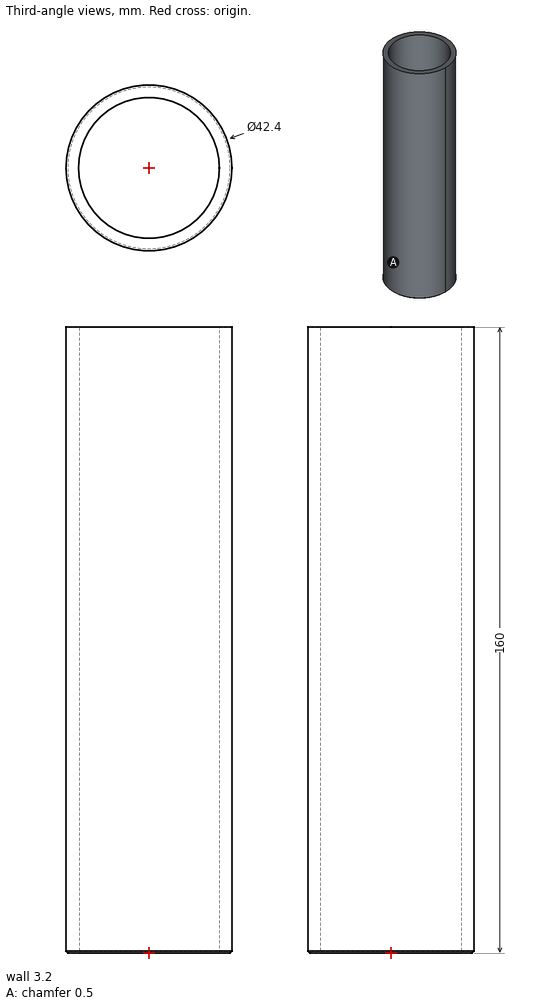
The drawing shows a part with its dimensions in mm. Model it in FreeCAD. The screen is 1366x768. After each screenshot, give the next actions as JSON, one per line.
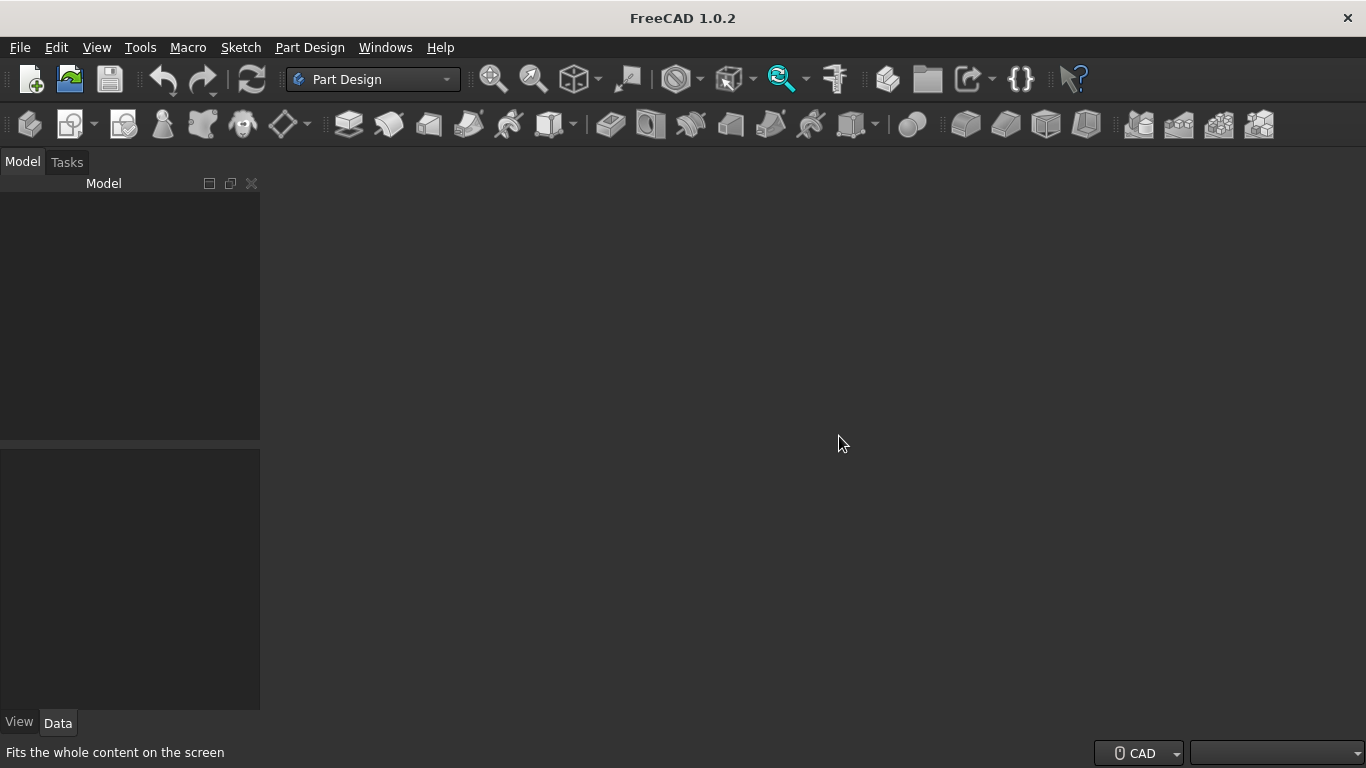
{"action": "left_click", "coordinate": [30, 80]}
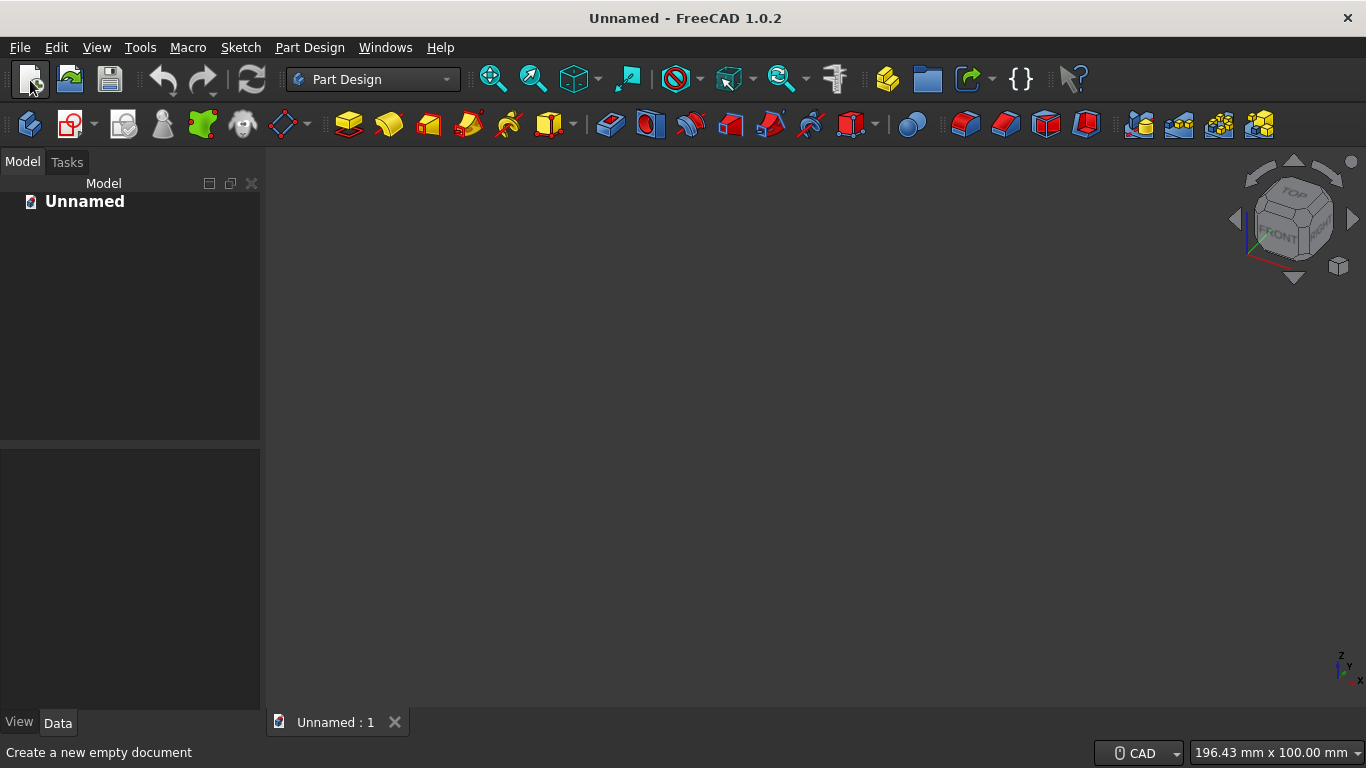
{"action": "left_click", "coordinate": [70, 124]}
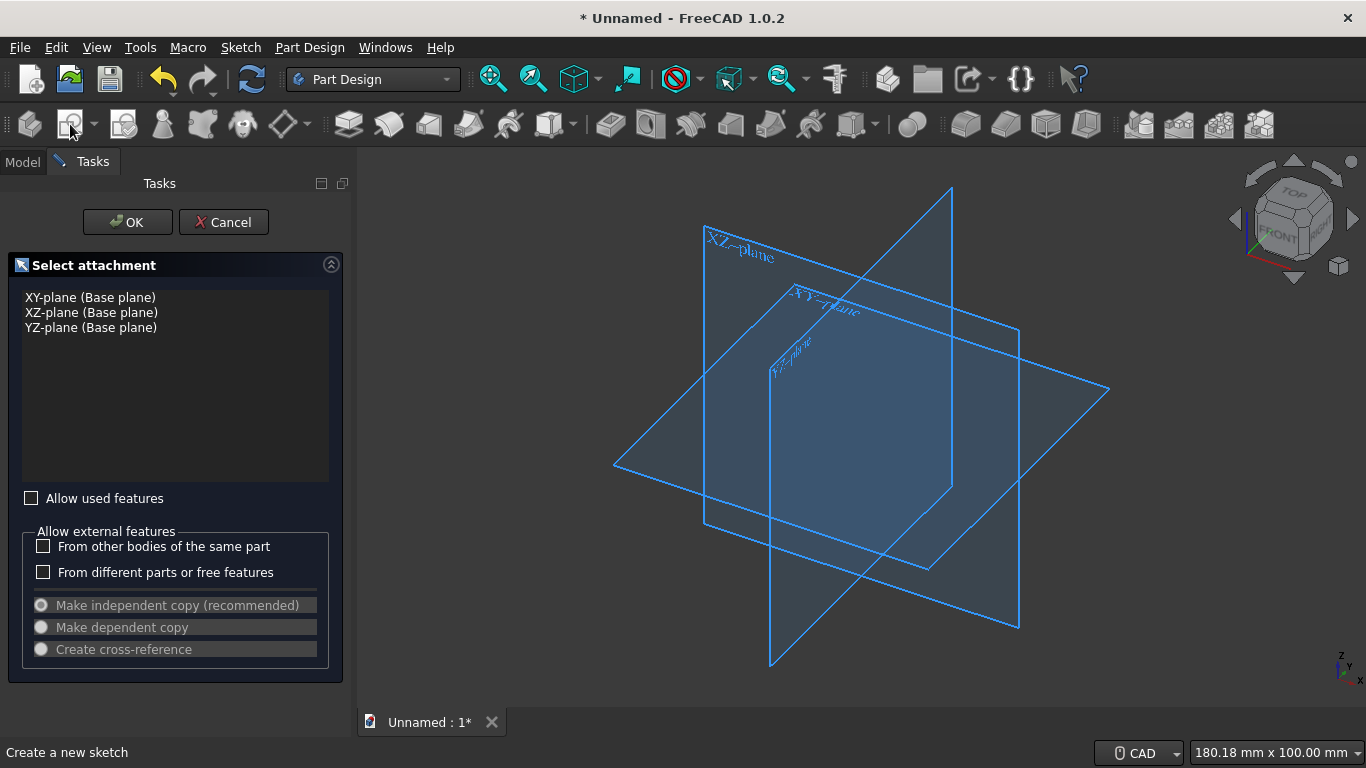
{"action": "left_click", "coordinate": [82, 298]}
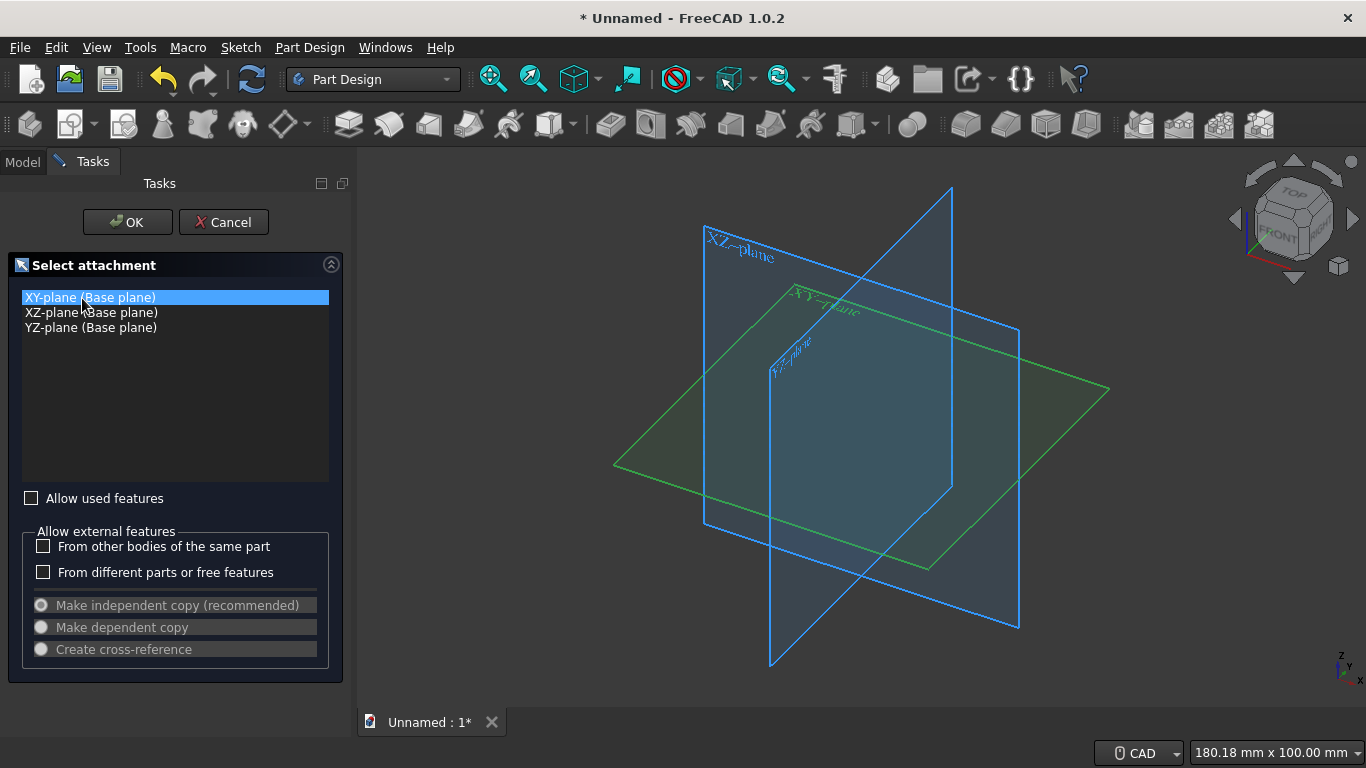
{"action": "left_click", "coordinate": [128, 222]}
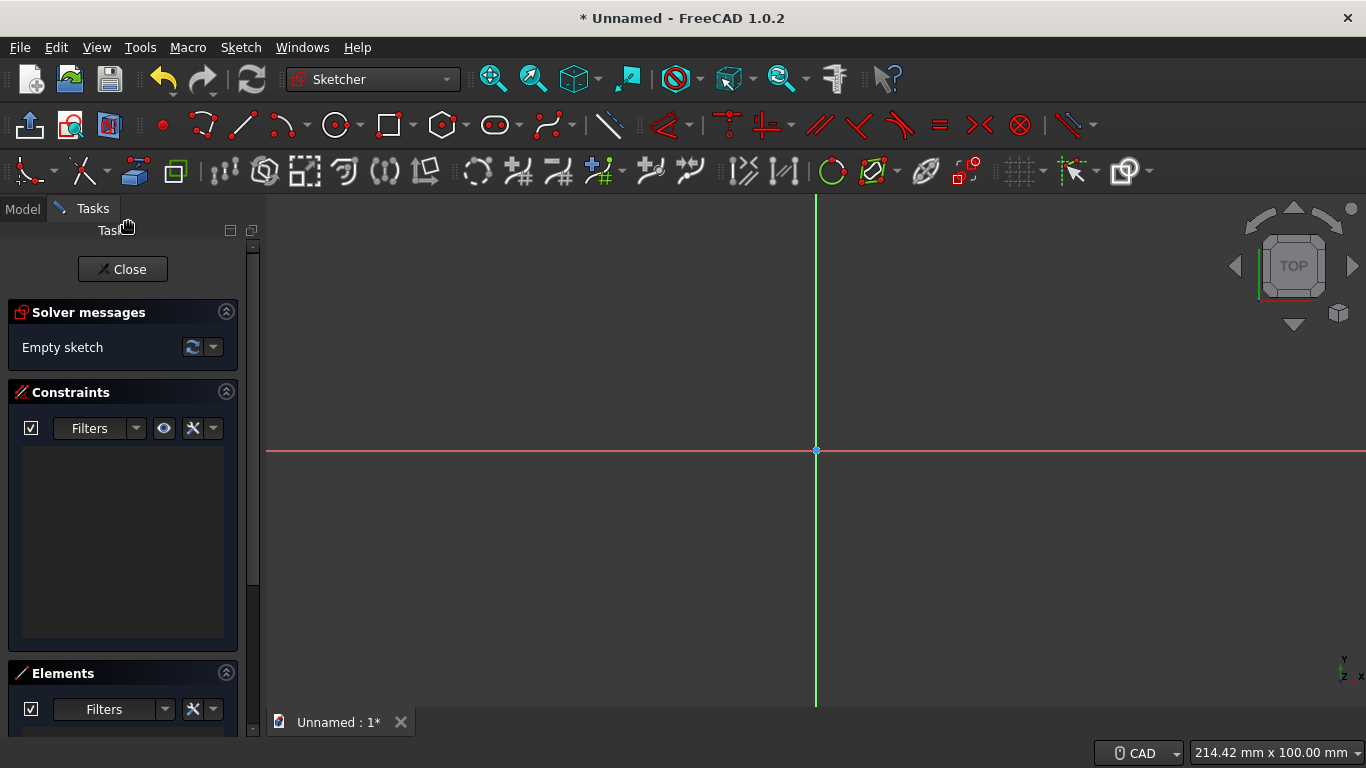
{"action": "scroll", "coordinate": [955, 451], "scroll_direction": "up", "scroll_amount": 2}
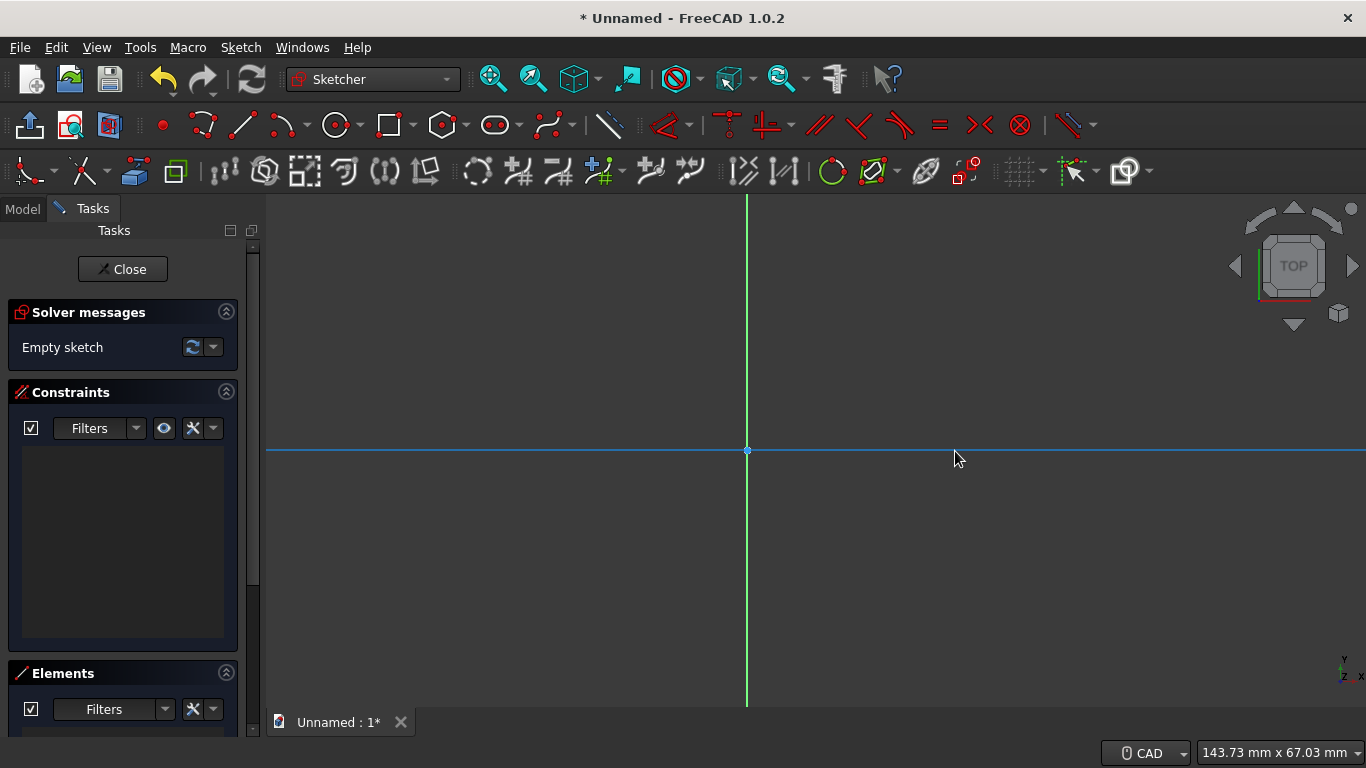
{"action": "left_click", "coordinate": [336, 126]}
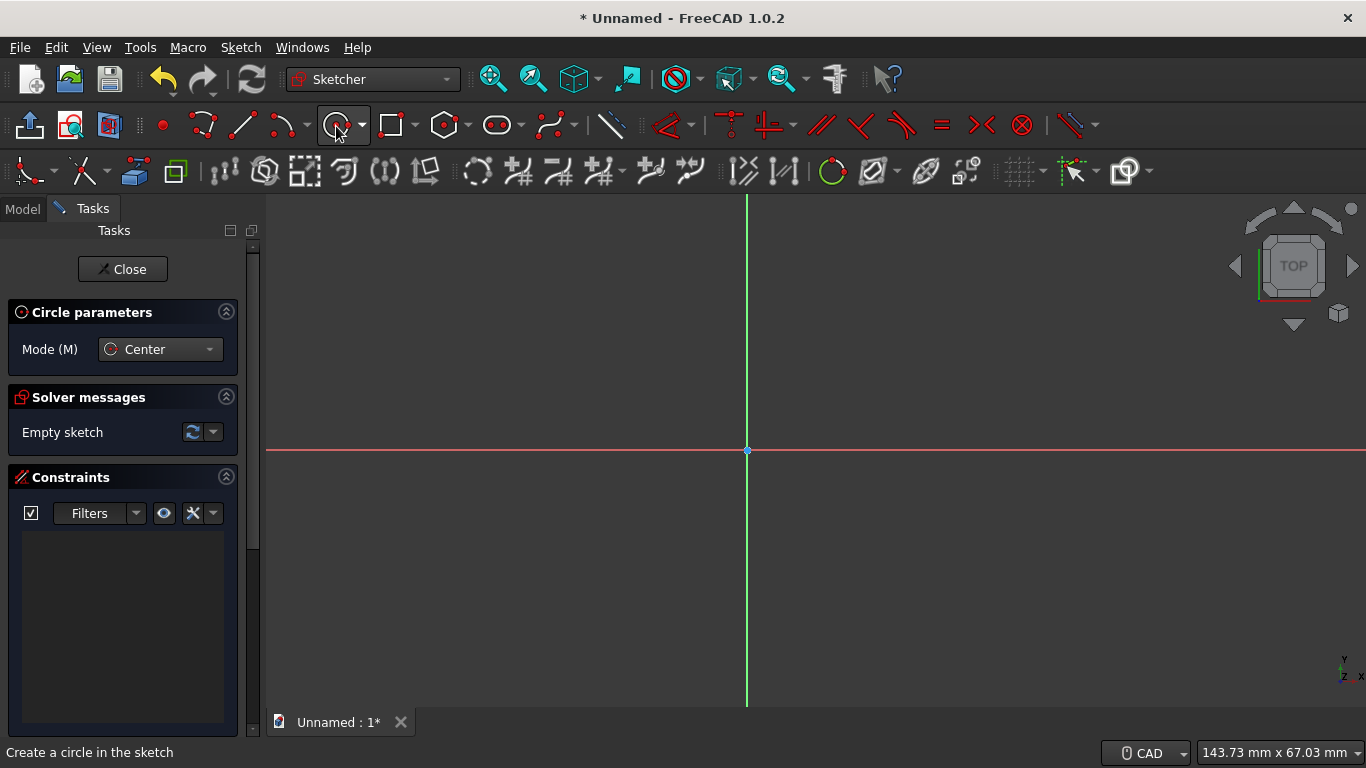
{"action": "left_click", "coordinate": [747, 450]}
{"action": "left_click", "coordinate": [862, 335]}
{"action": "key", "text": "Escape"}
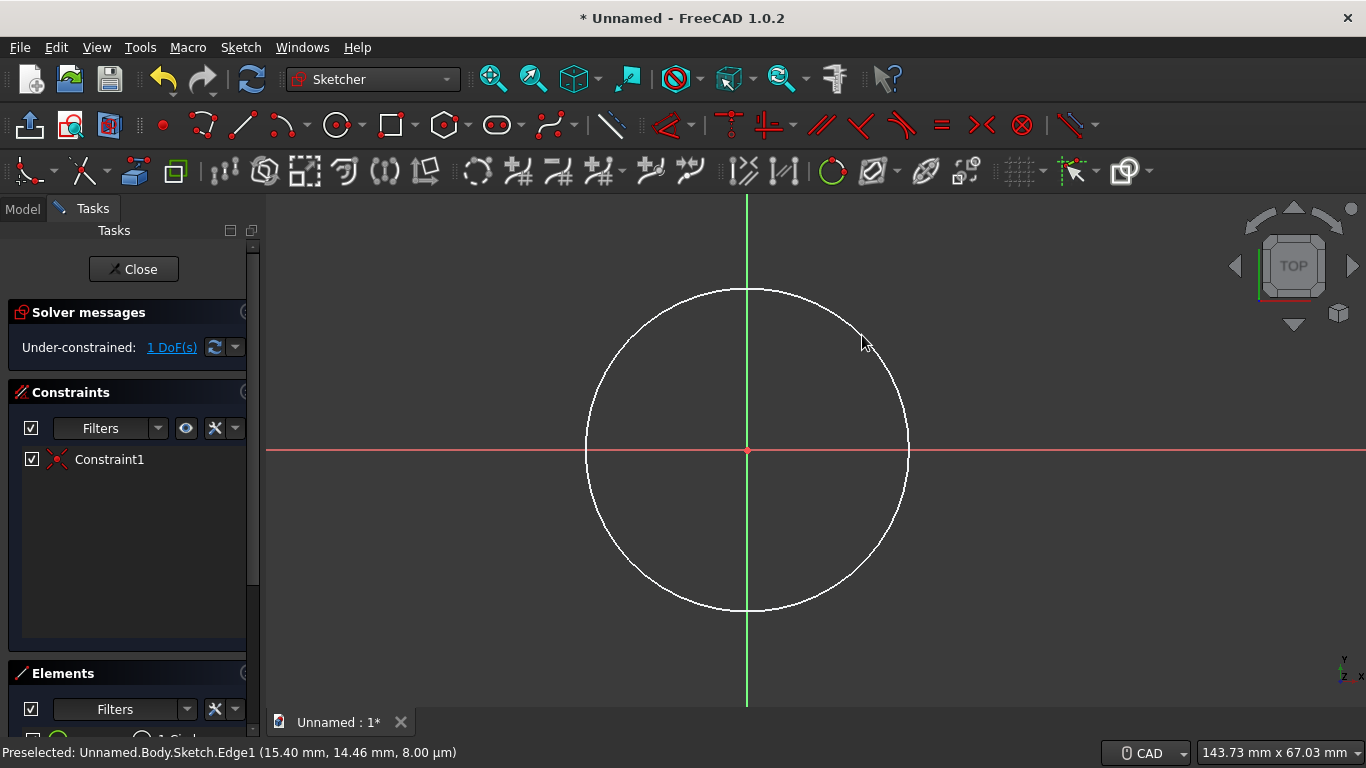
{"action": "left_click", "coordinate": [666, 126]}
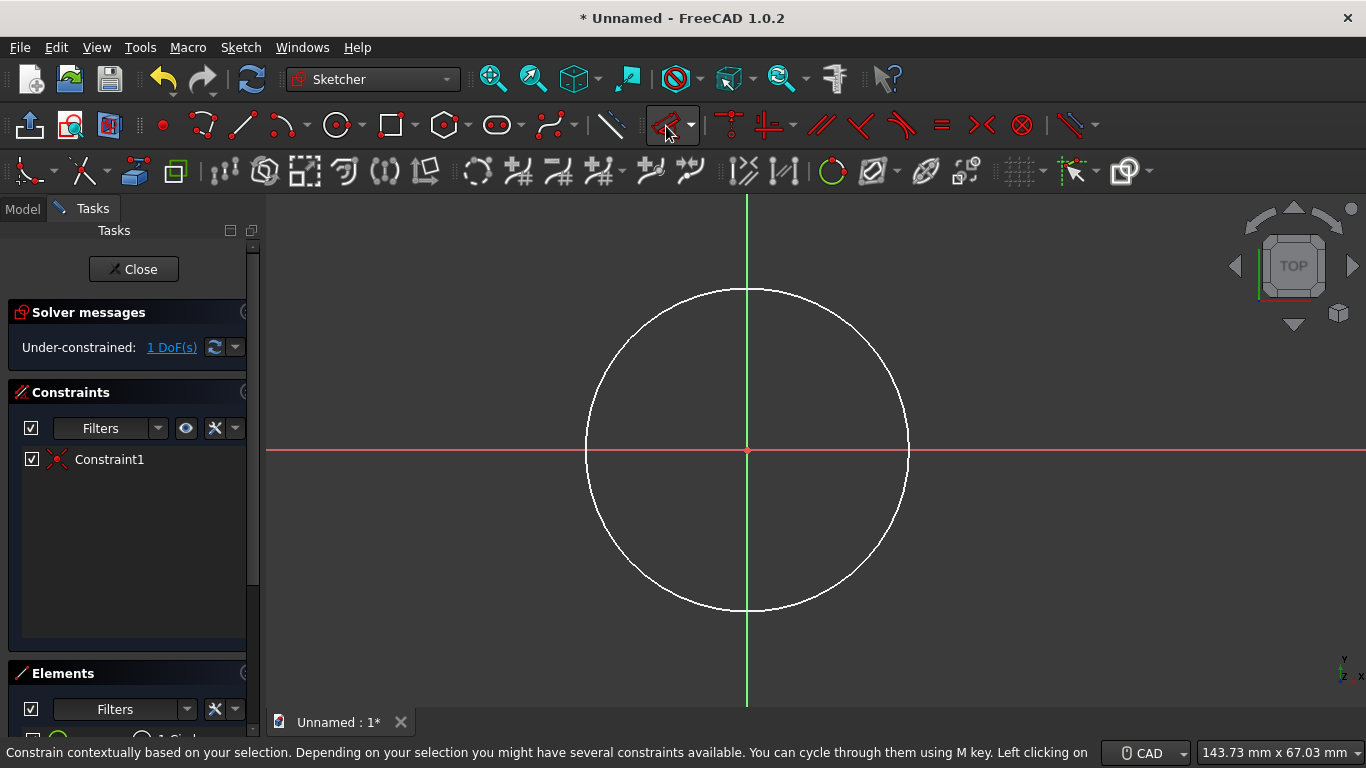
{"action": "left_click", "coordinate": [861, 335]}
{"action": "left_click", "coordinate": [883, 312]}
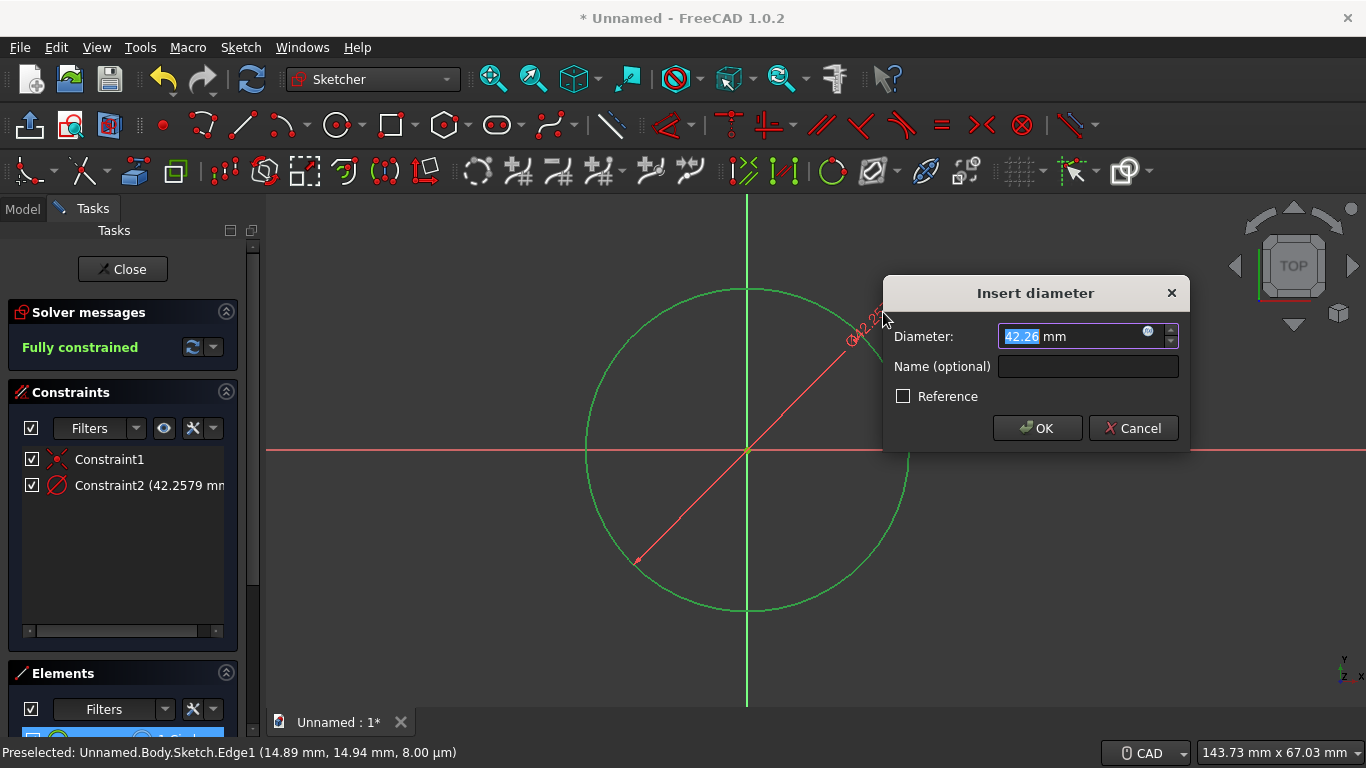
{"action": "type", "text": "42.4"}
{"action": "key", "text": "Return"}
{"action": "key", "text": "Escape"}